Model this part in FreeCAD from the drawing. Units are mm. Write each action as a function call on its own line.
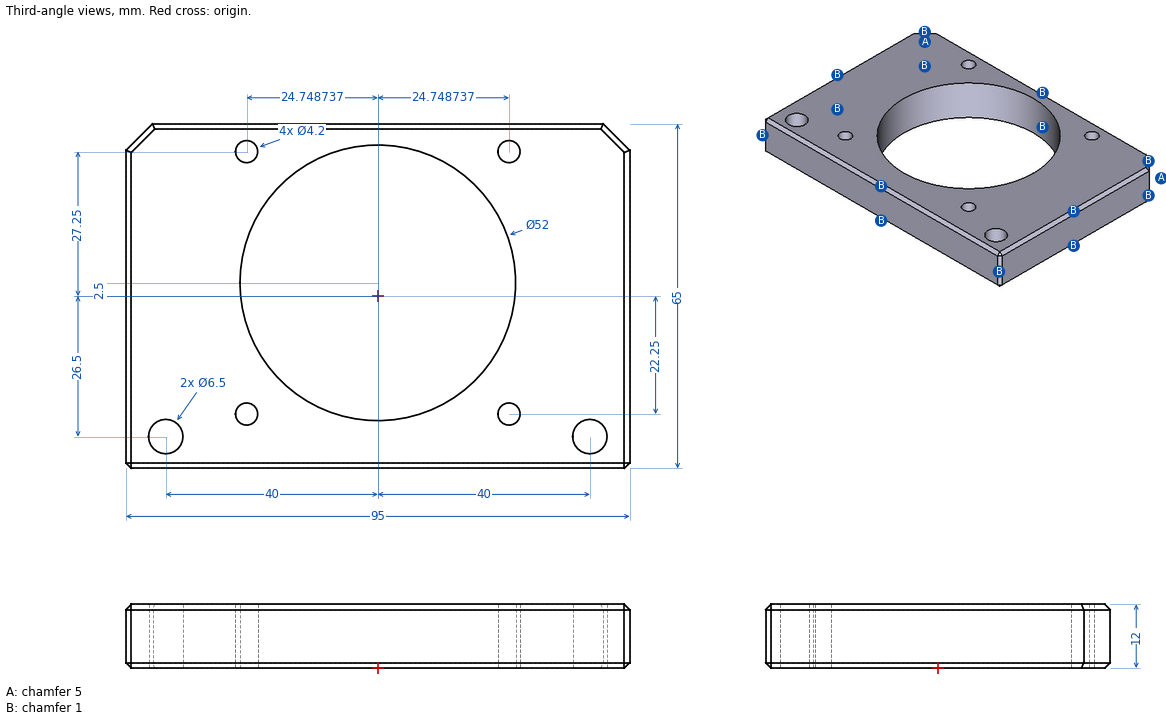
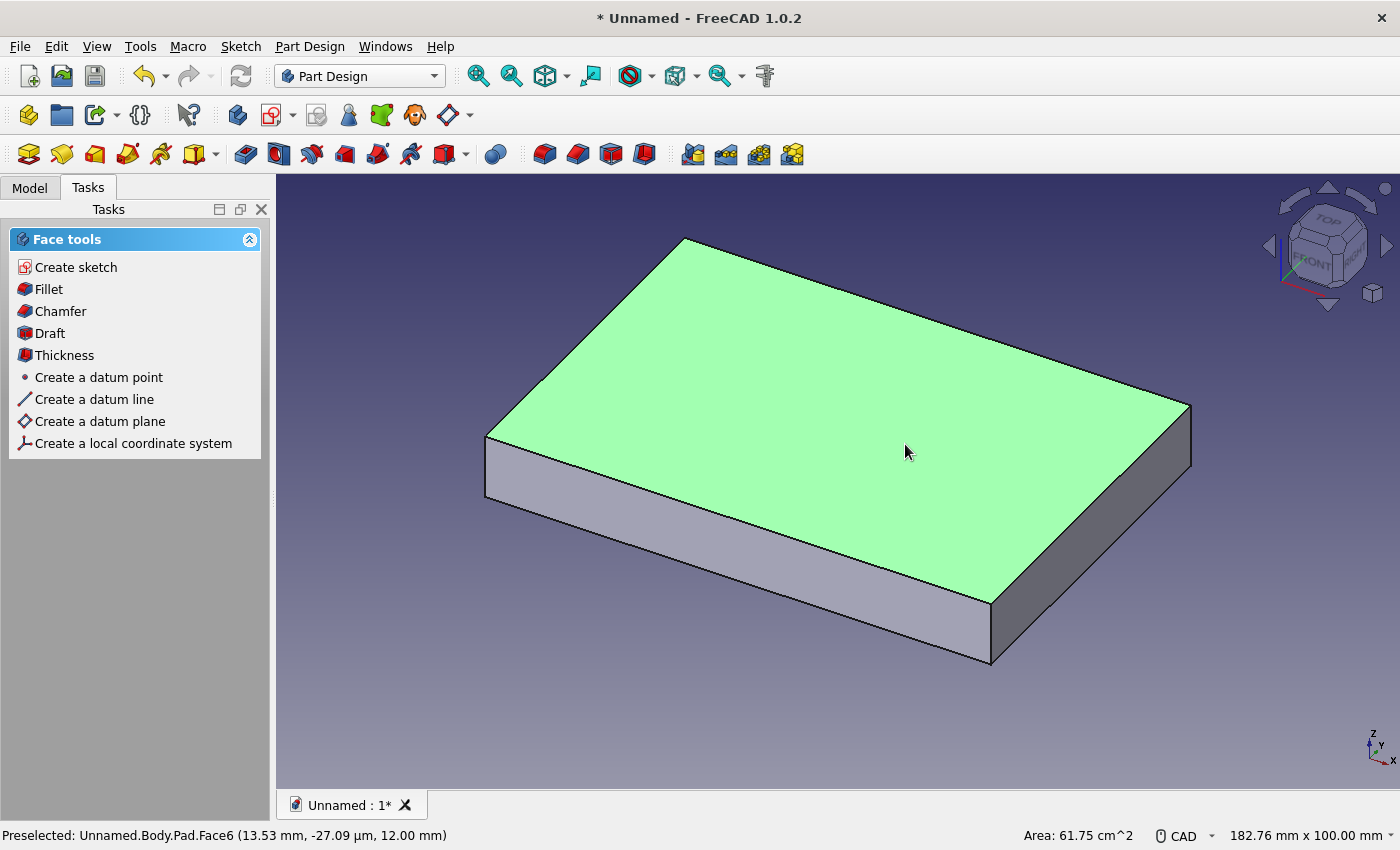
click(270, 116)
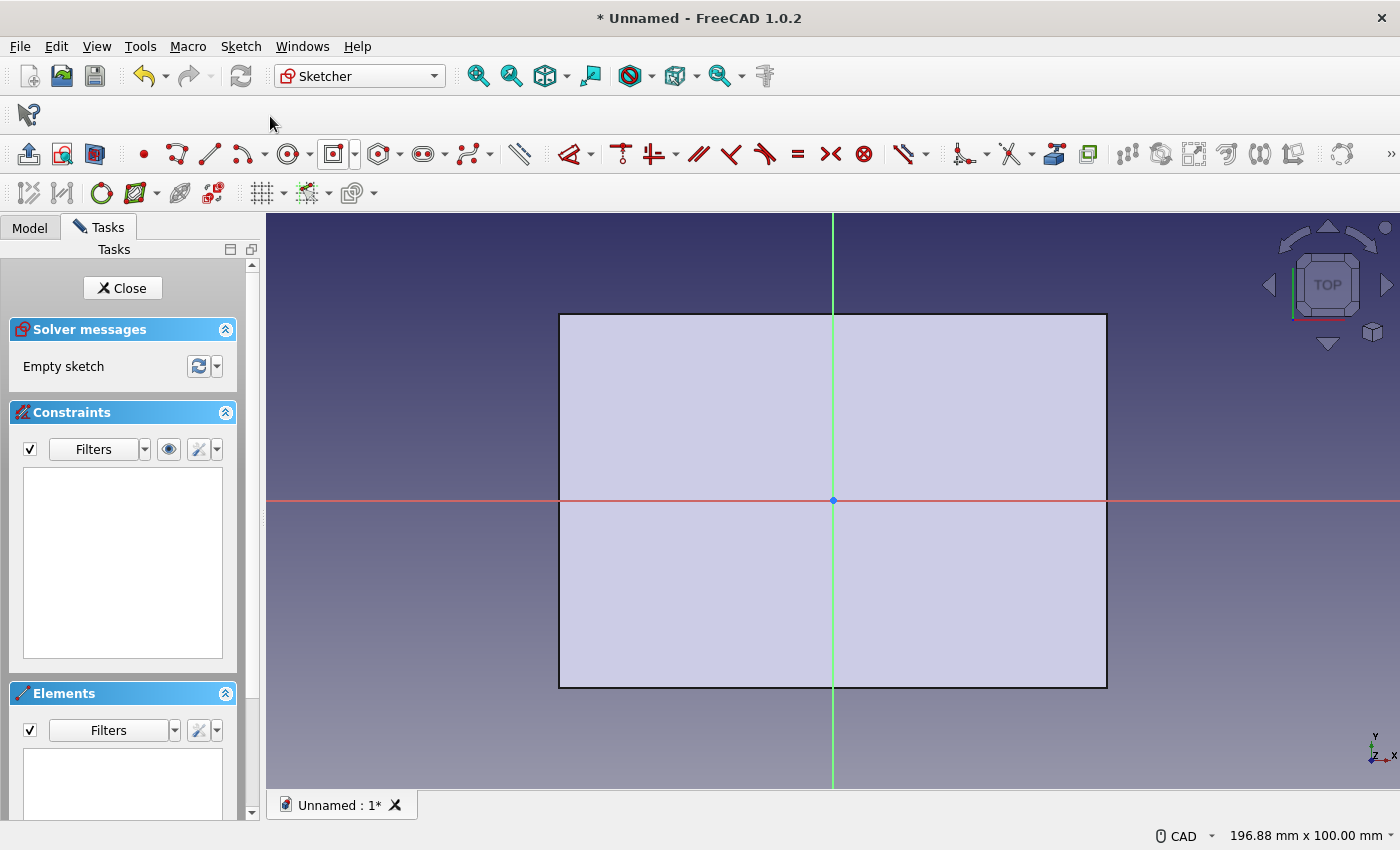
key(g)
key(c)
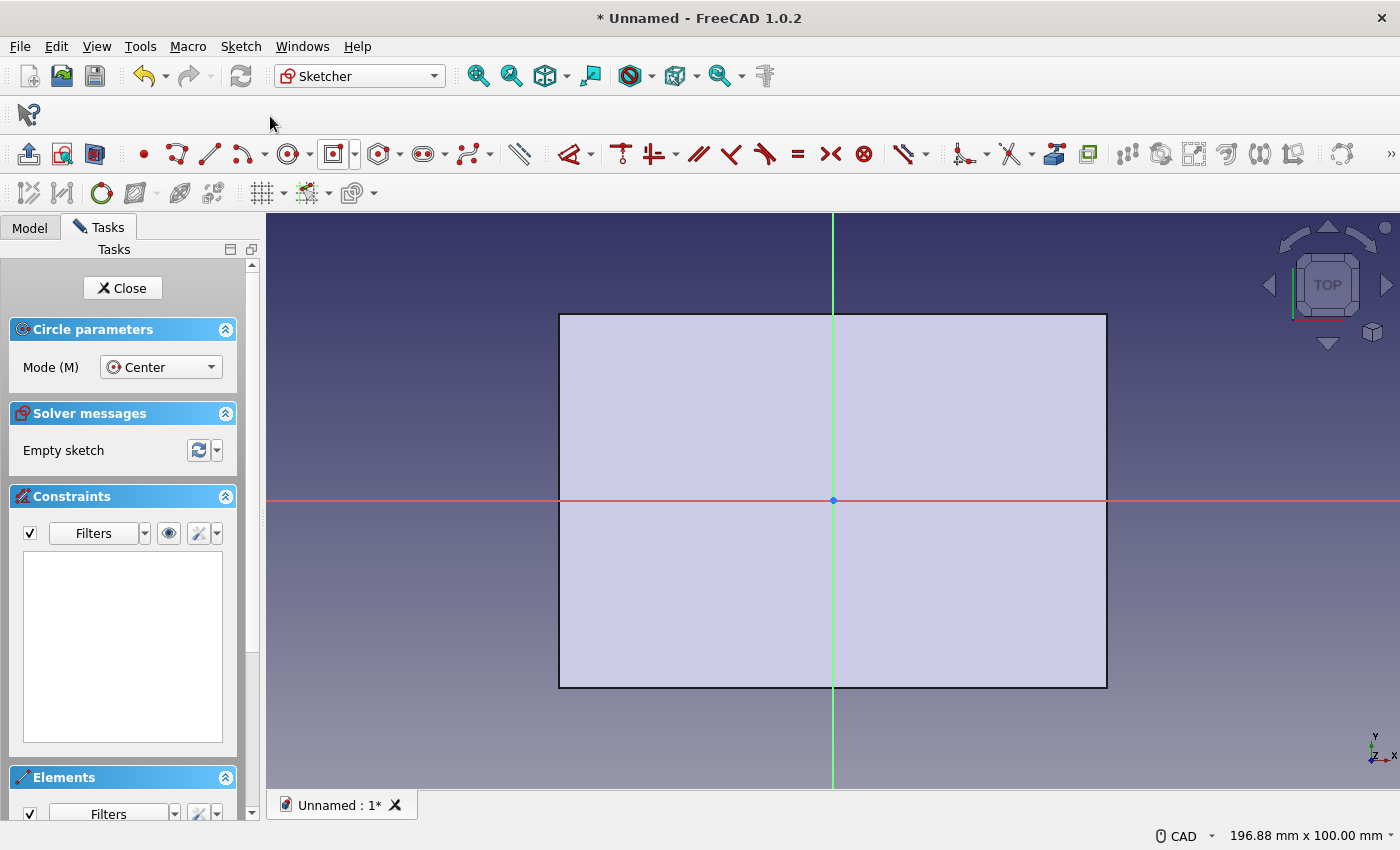
click(603, 654)
click(616, 640)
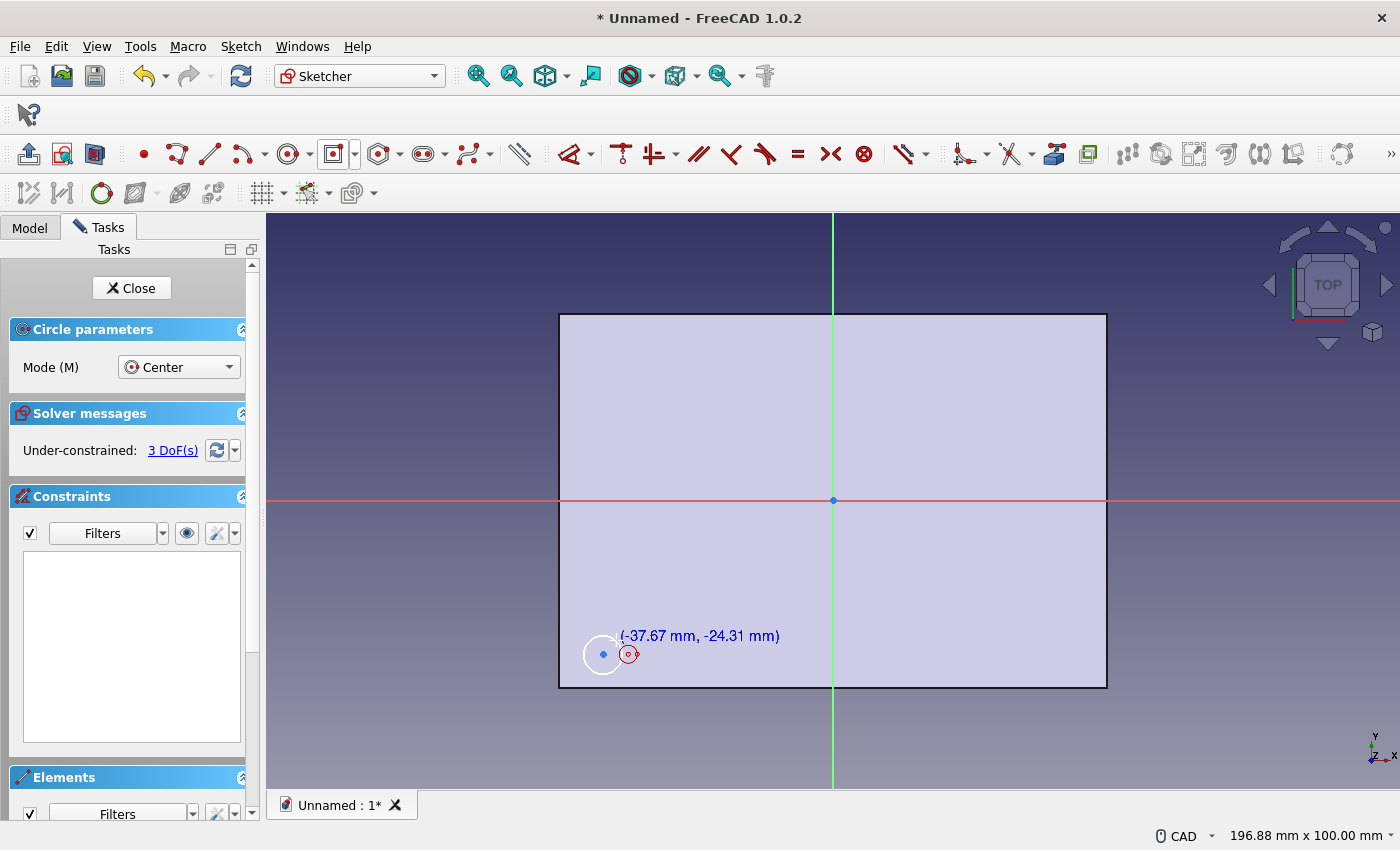
click(1063, 654)
click(1077, 640)
key(Escape)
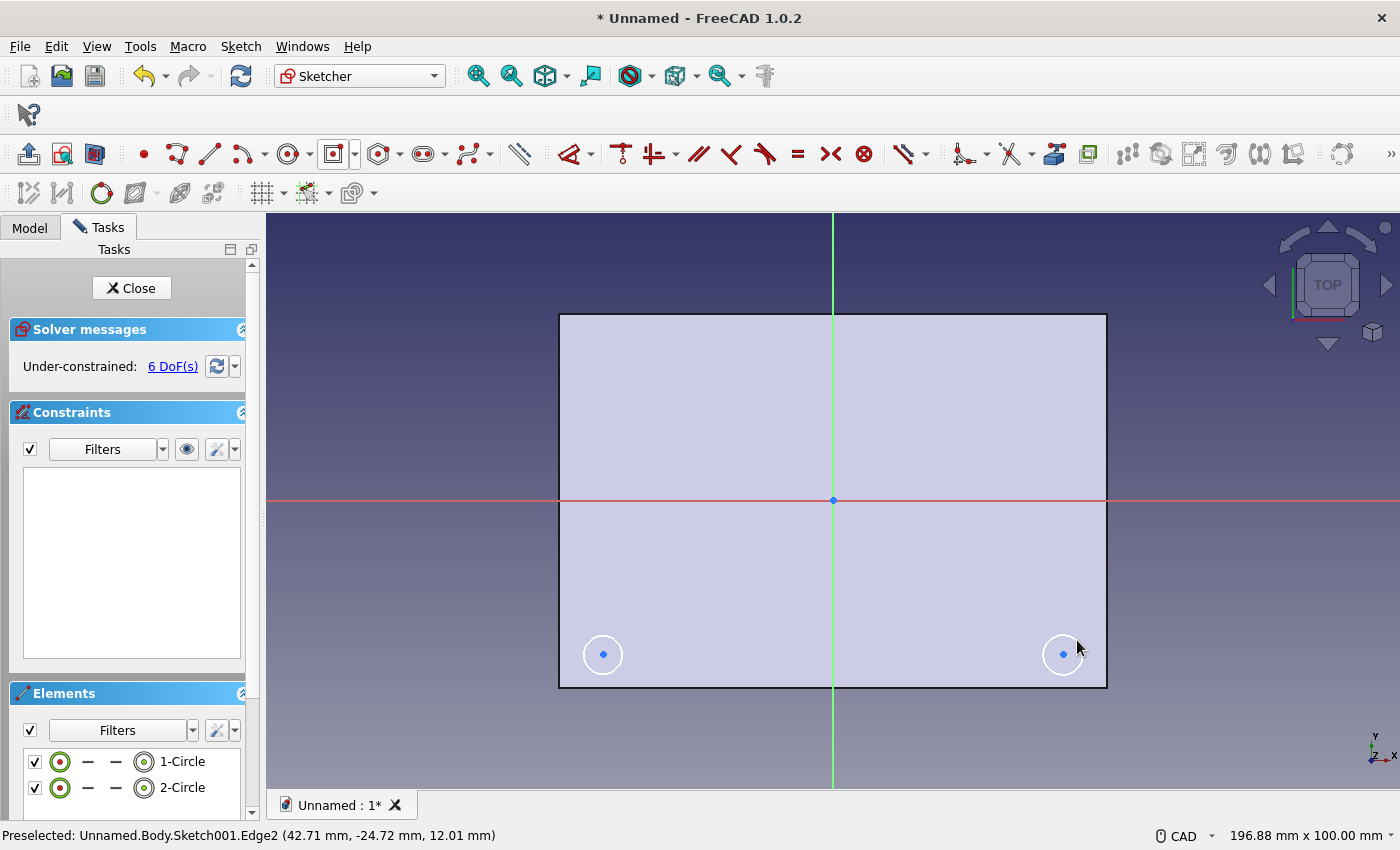
click(616, 641)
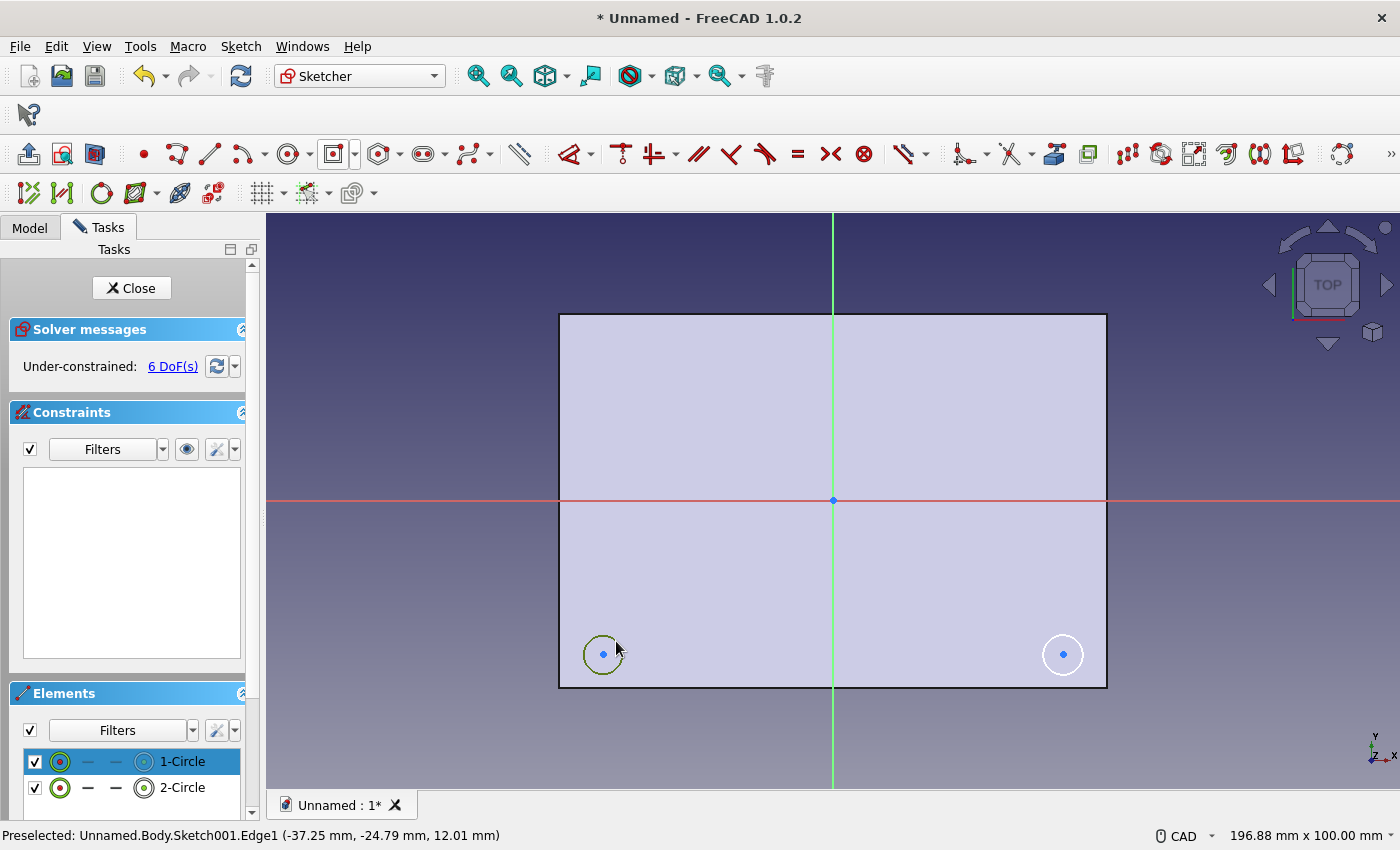
click(1077, 641)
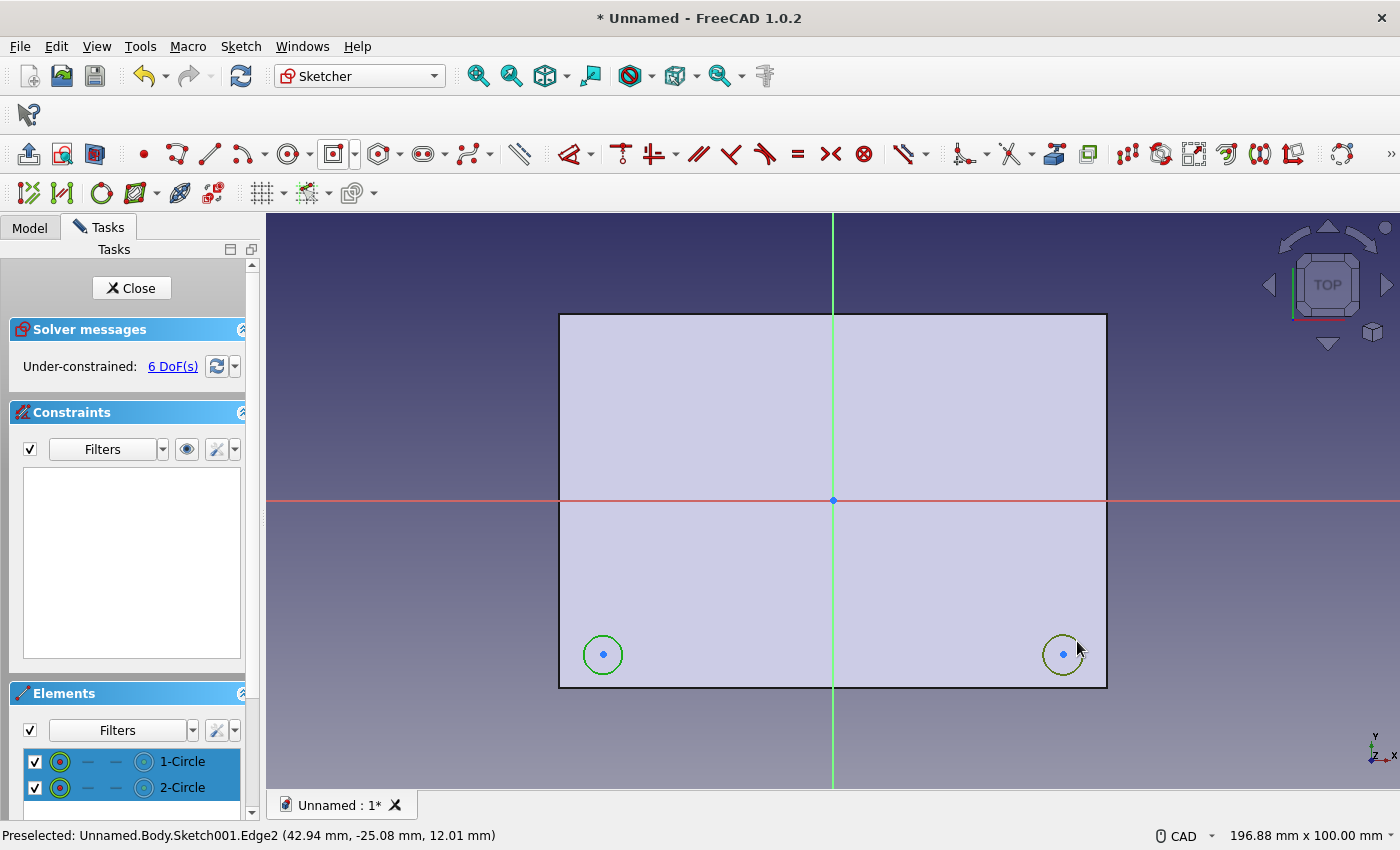
key(e)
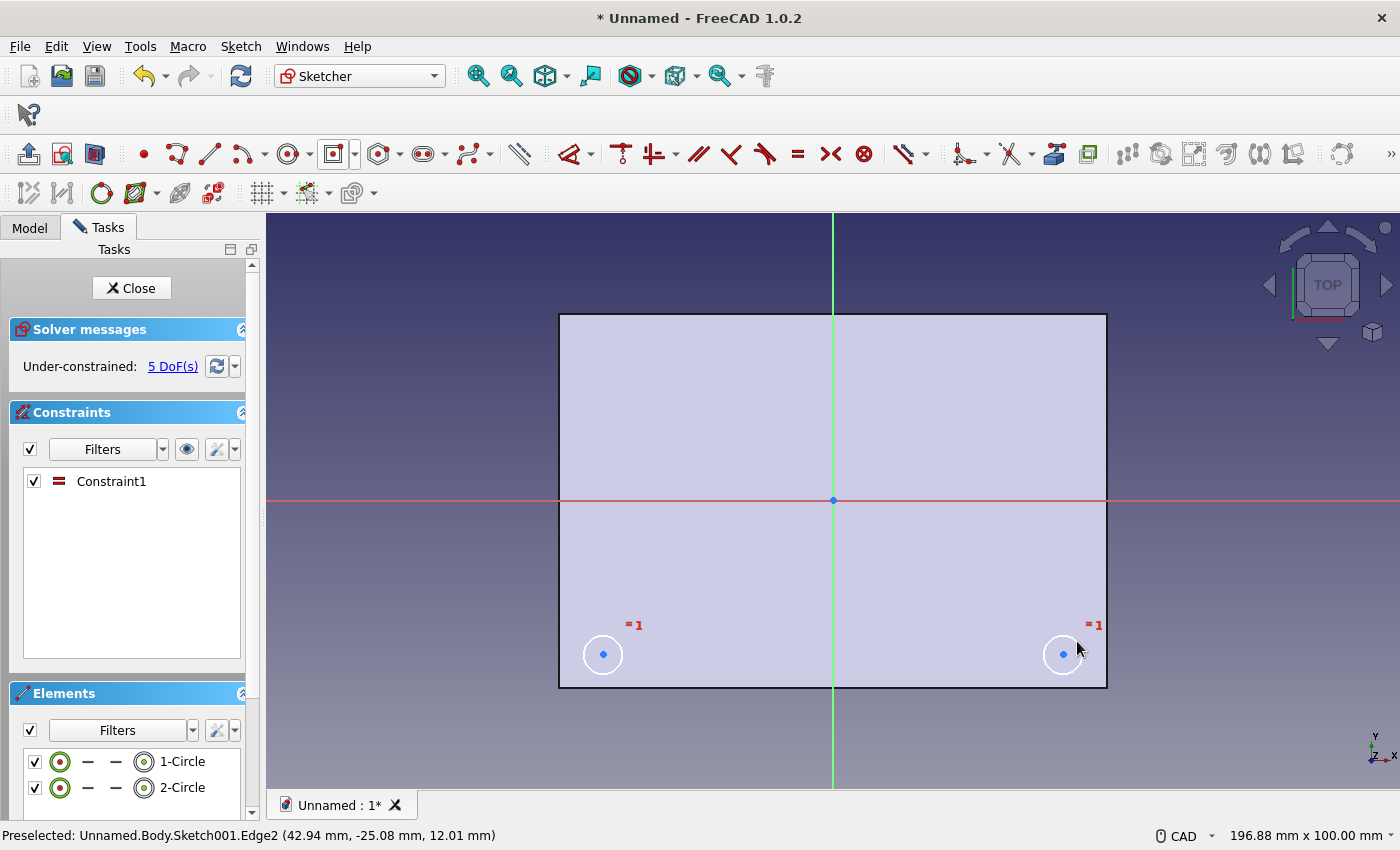
click(603, 655)